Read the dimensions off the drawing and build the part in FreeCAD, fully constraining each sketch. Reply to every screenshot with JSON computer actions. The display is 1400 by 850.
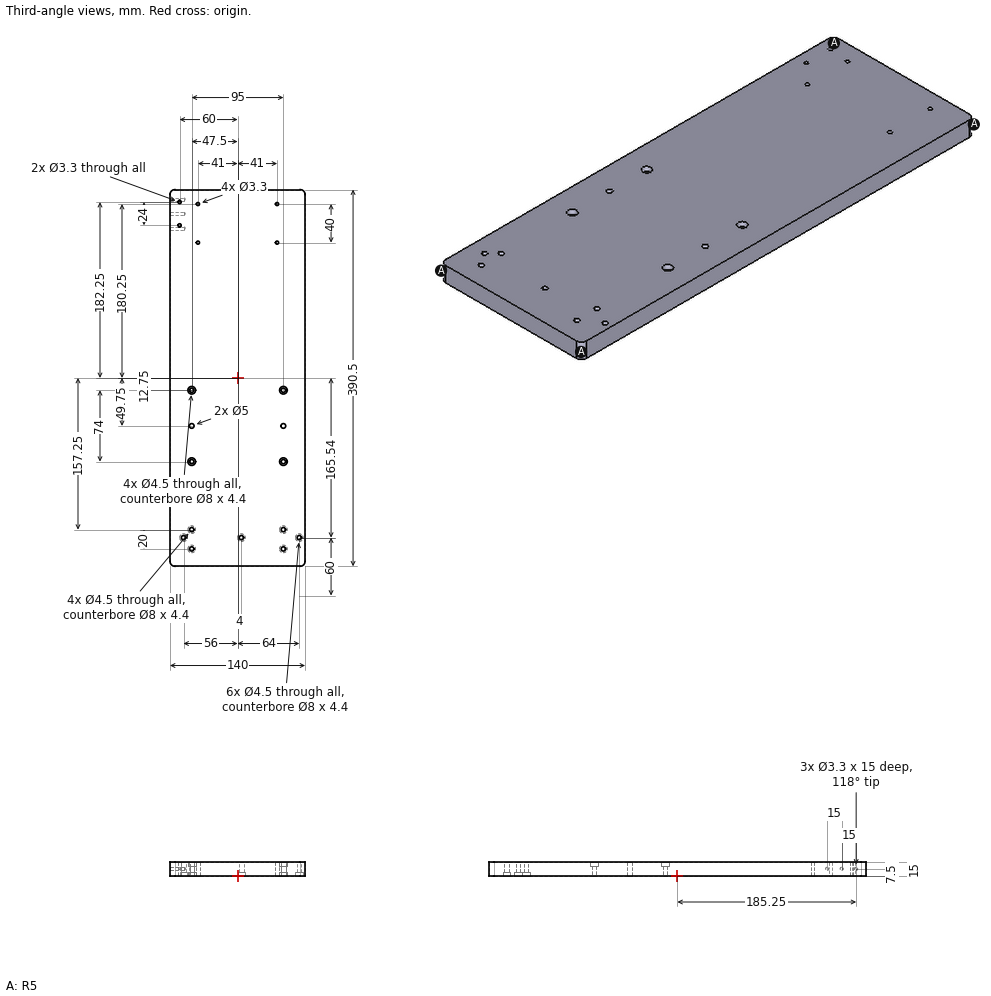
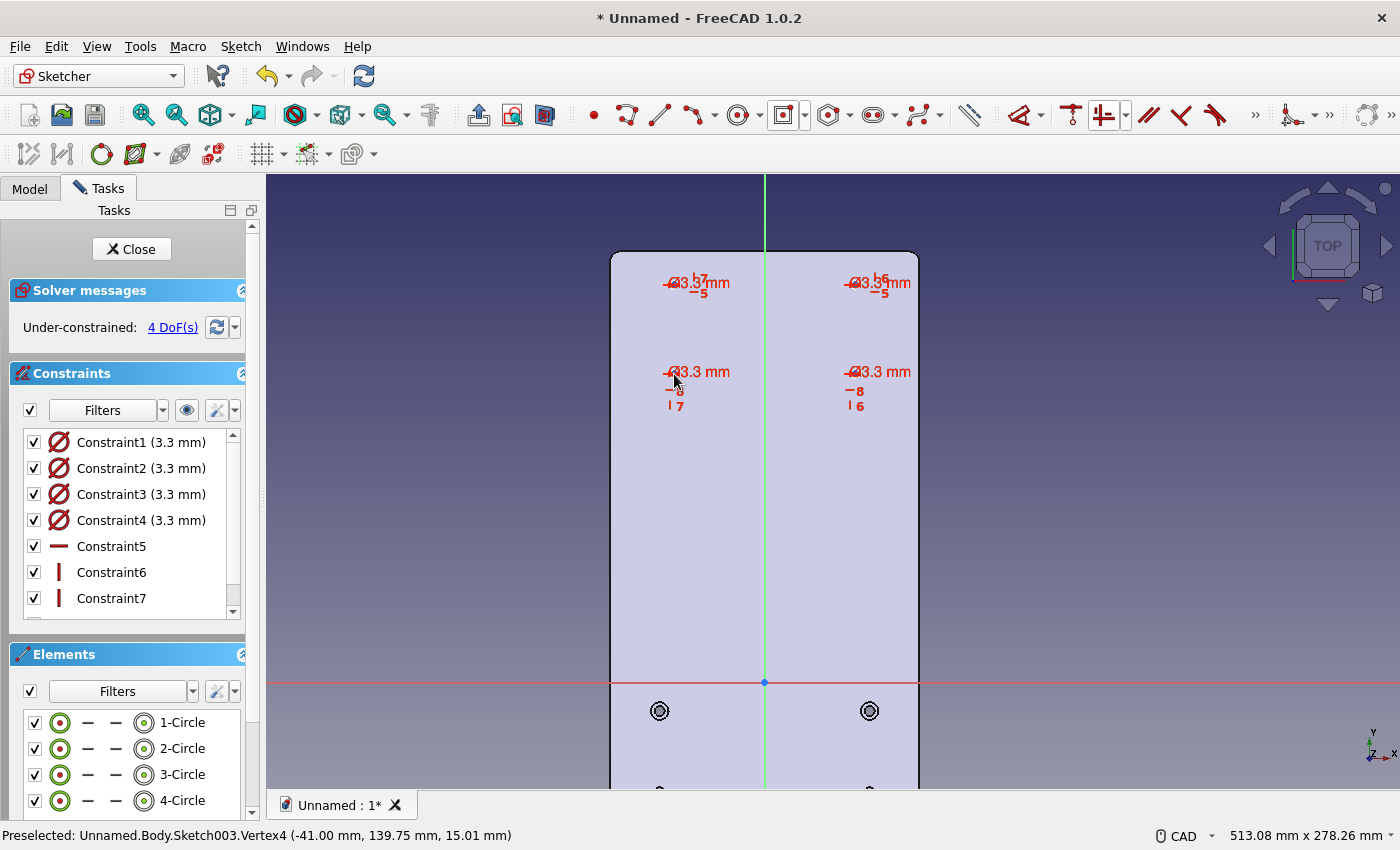
{"action": "left_click", "coordinate": [1018, 116]}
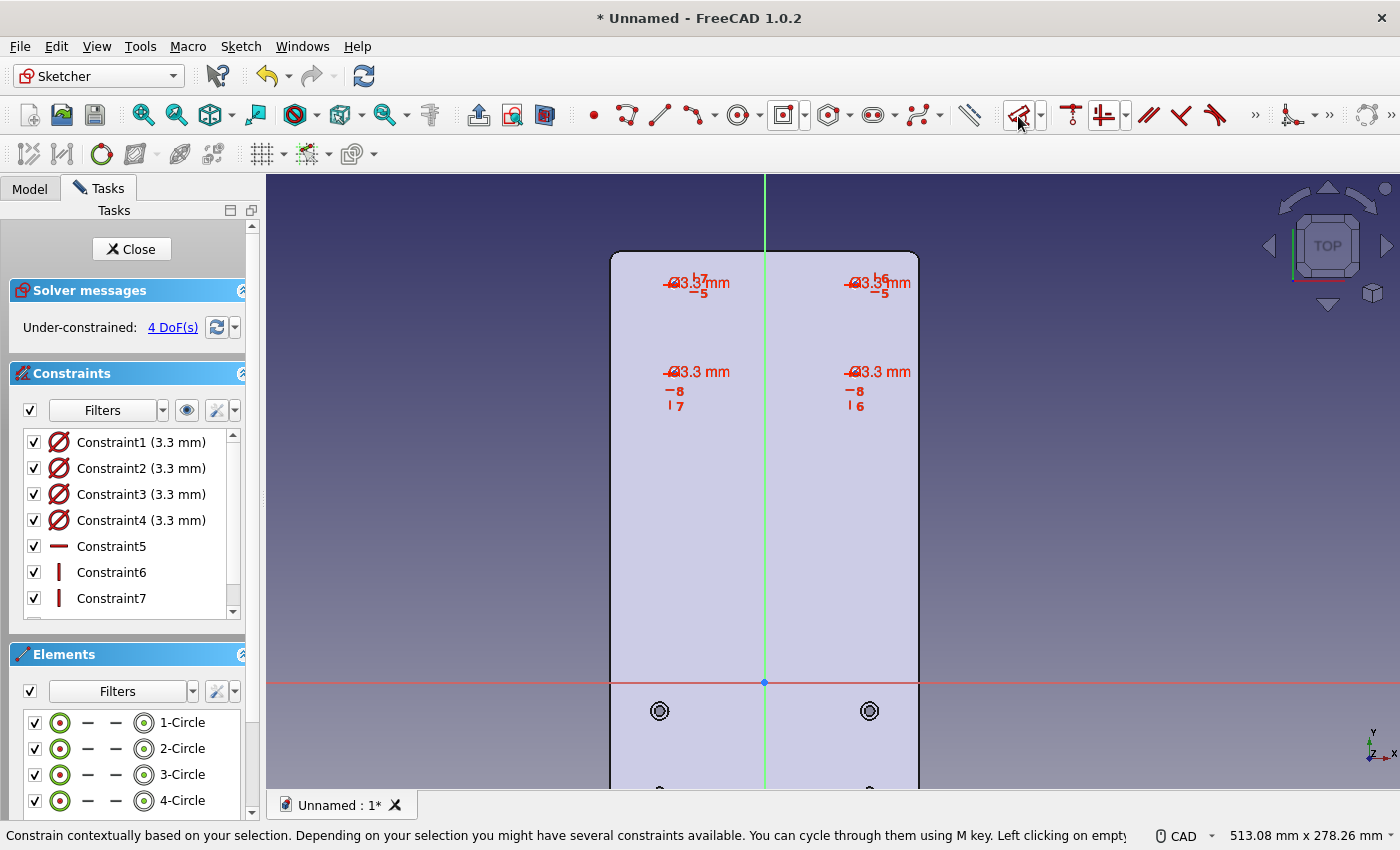
{"action": "left_click", "coordinate": [674, 285]}
{"action": "left_click", "coordinate": [719, 717]}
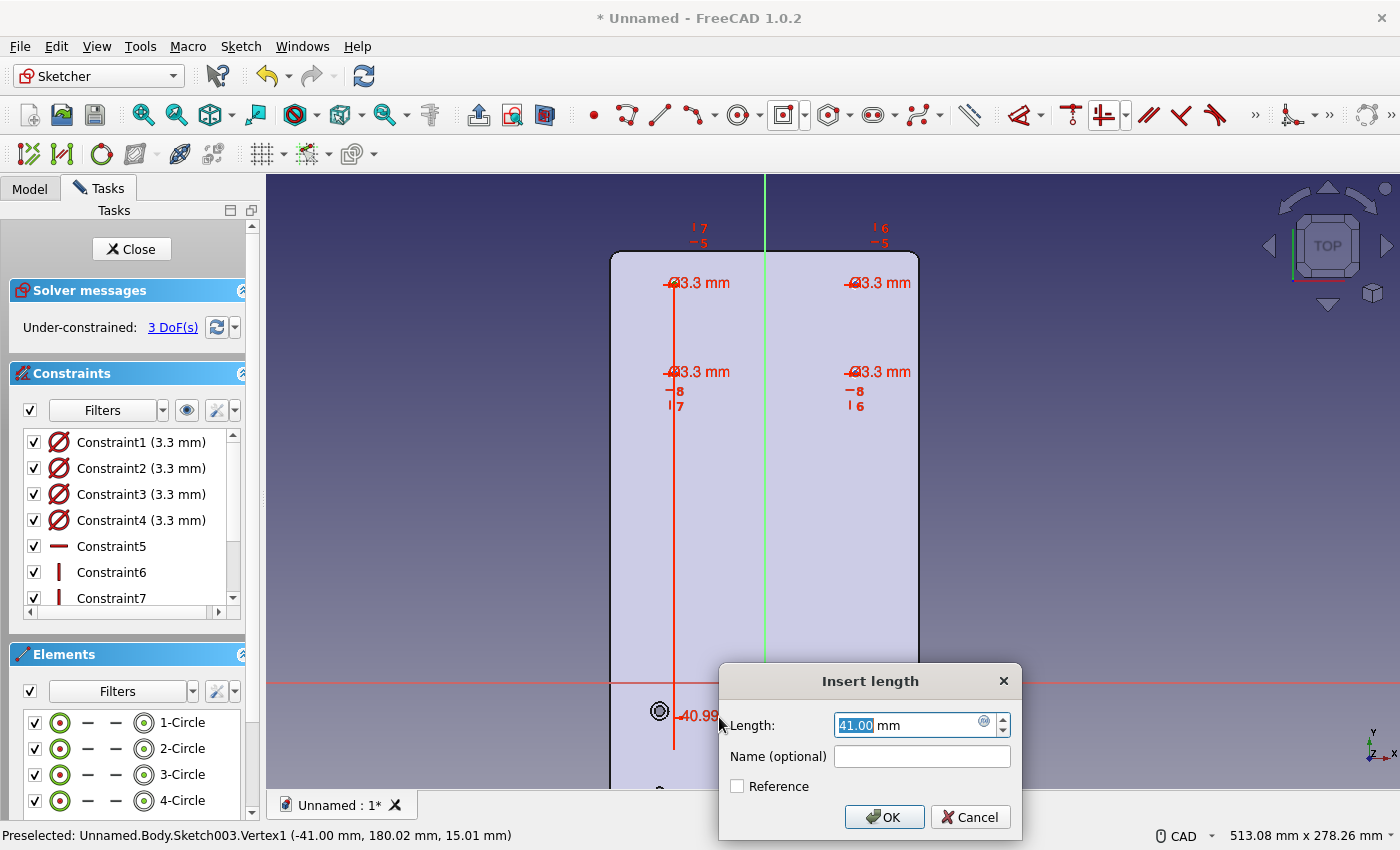
{"action": "type", "text": "41"}
{"action": "key", "text": "Return"}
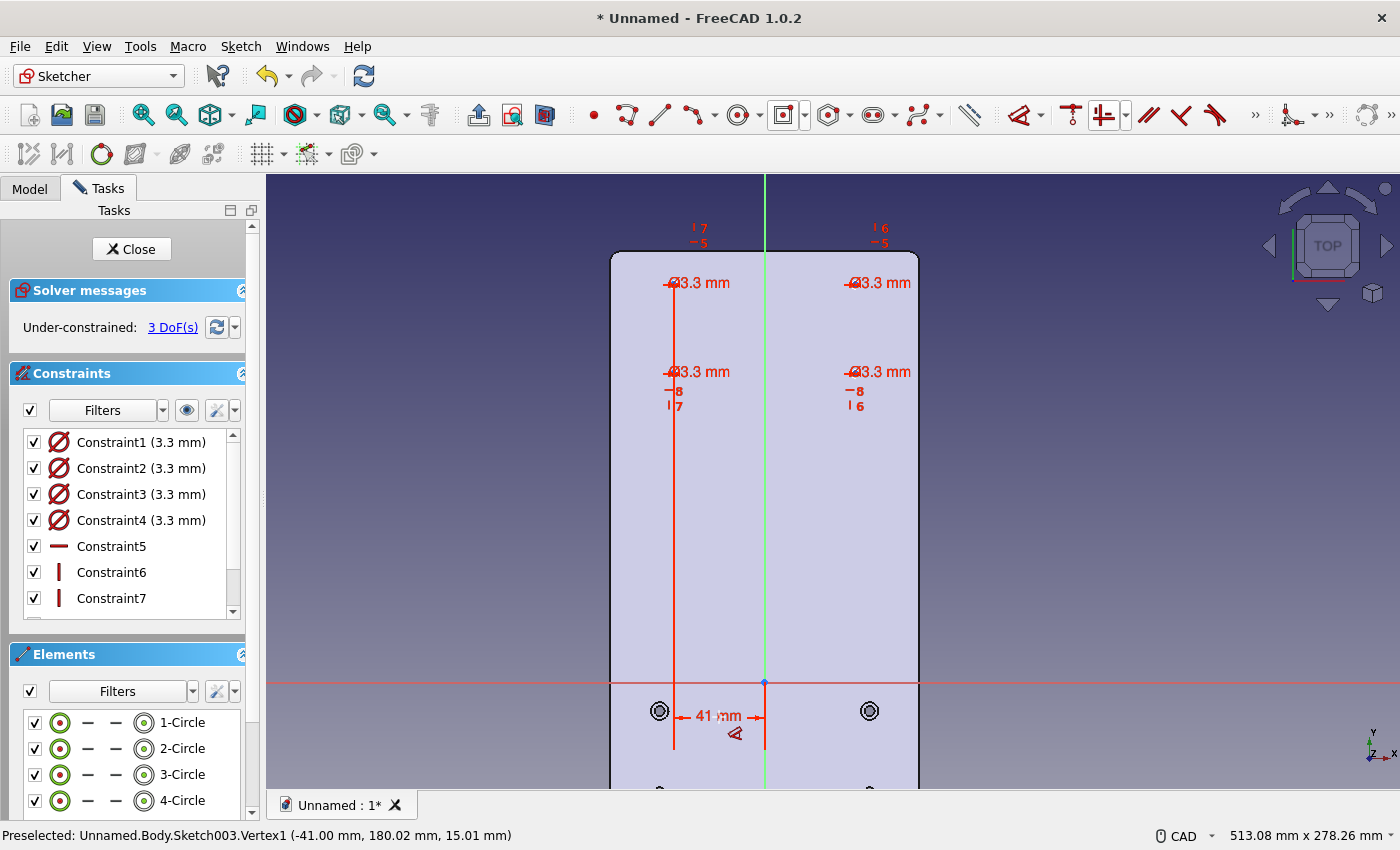
{"action": "left_click", "coordinate": [855, 285]}
{"action": "left_click", "coordinate": [810, 717]}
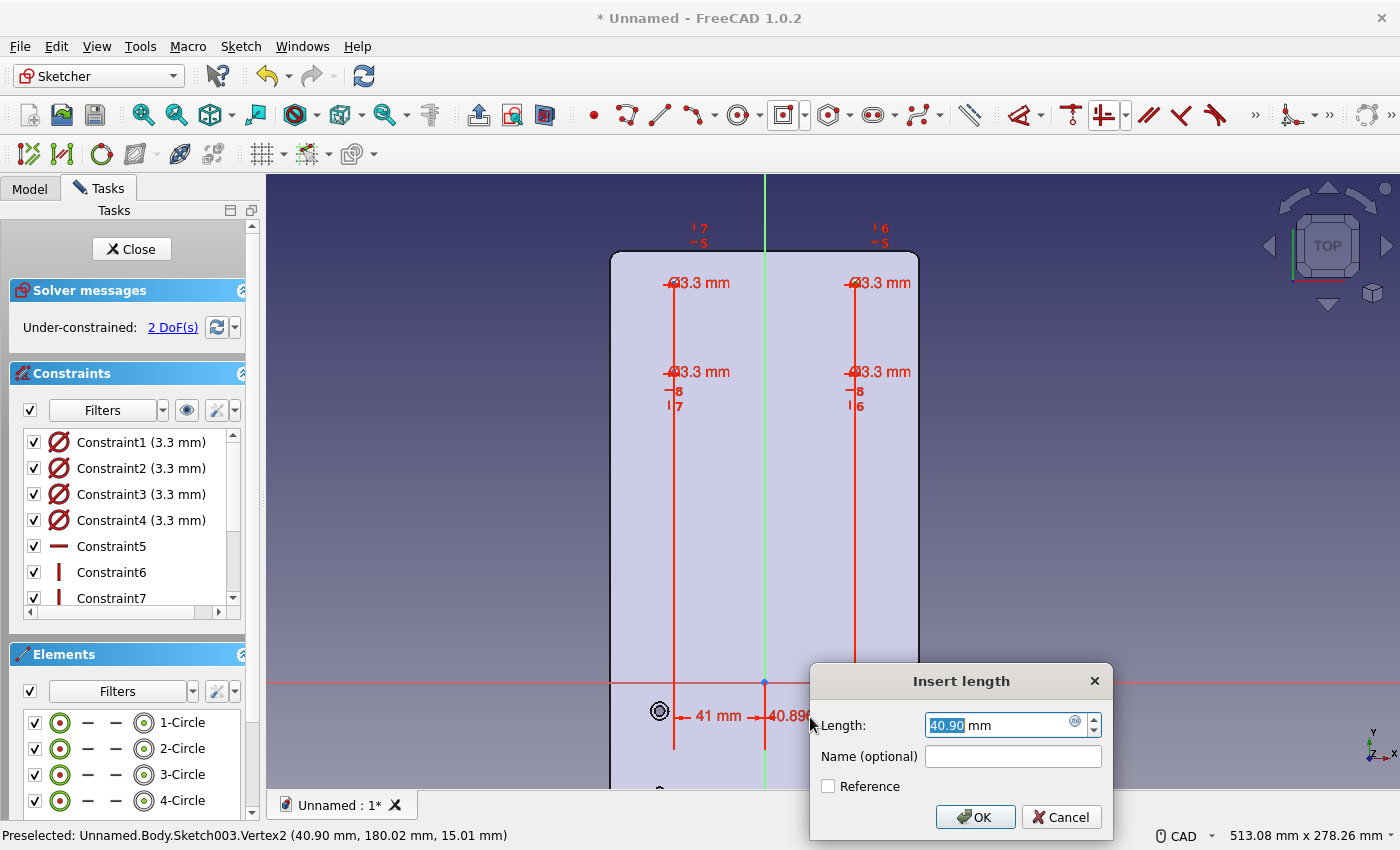
{"action": "type", "text": "41"}
{"action": "key", "text": "Return"}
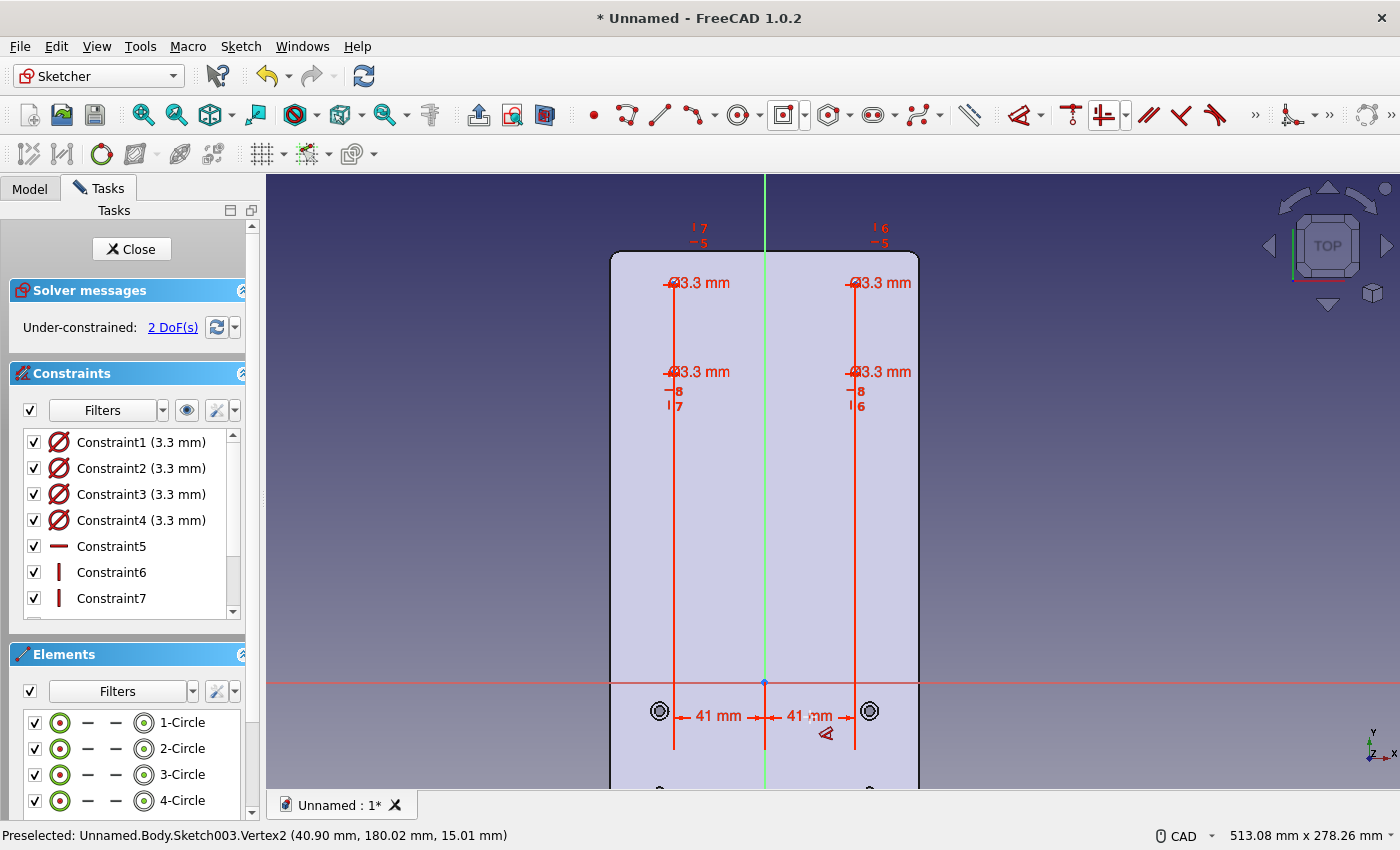
{"action": "left_click", "coordinate": [855, 285]}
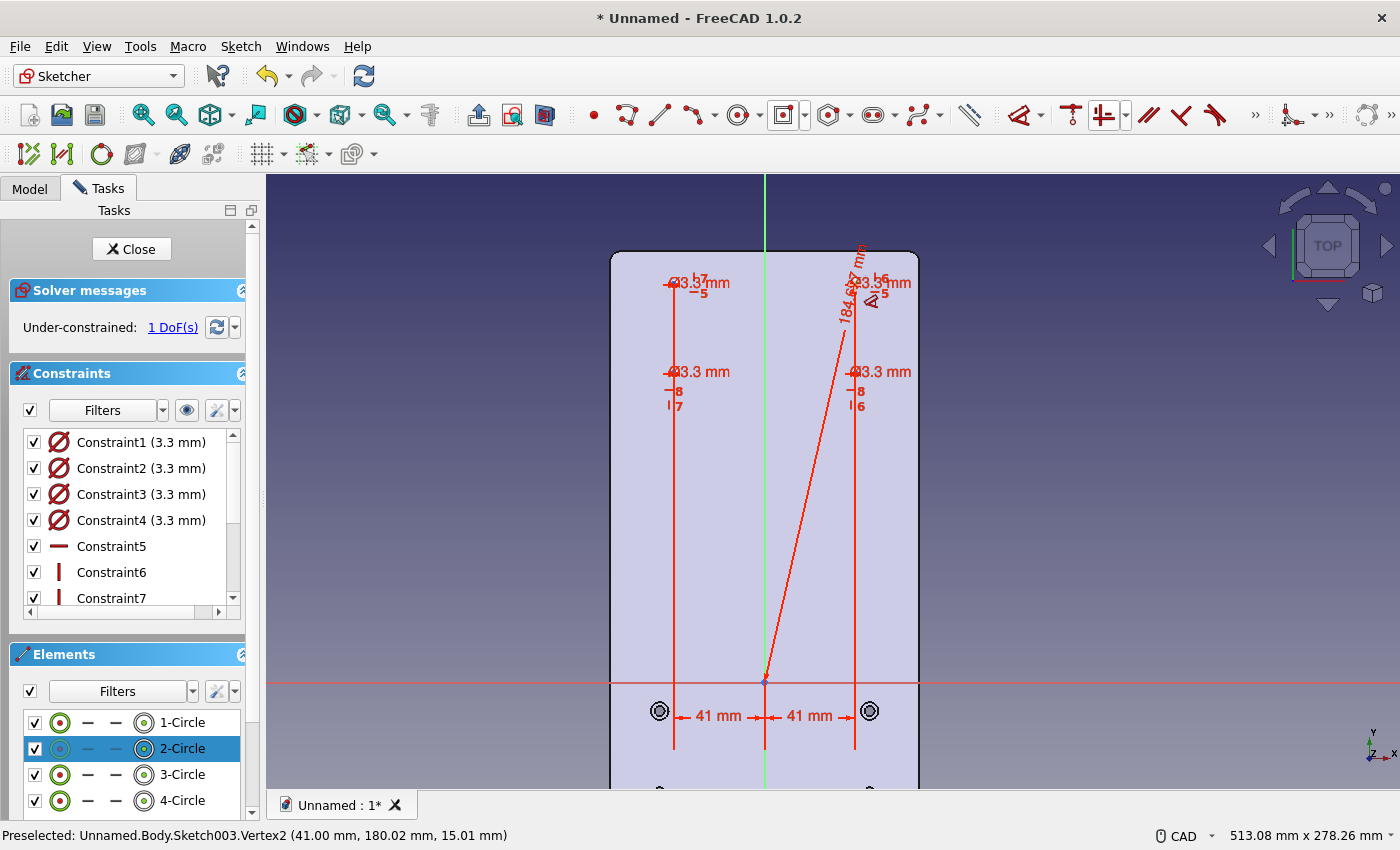
{"action": "left_click", "coordinate": [855, 374]}
{"action": "left_click", "coordinate": [889, 330]}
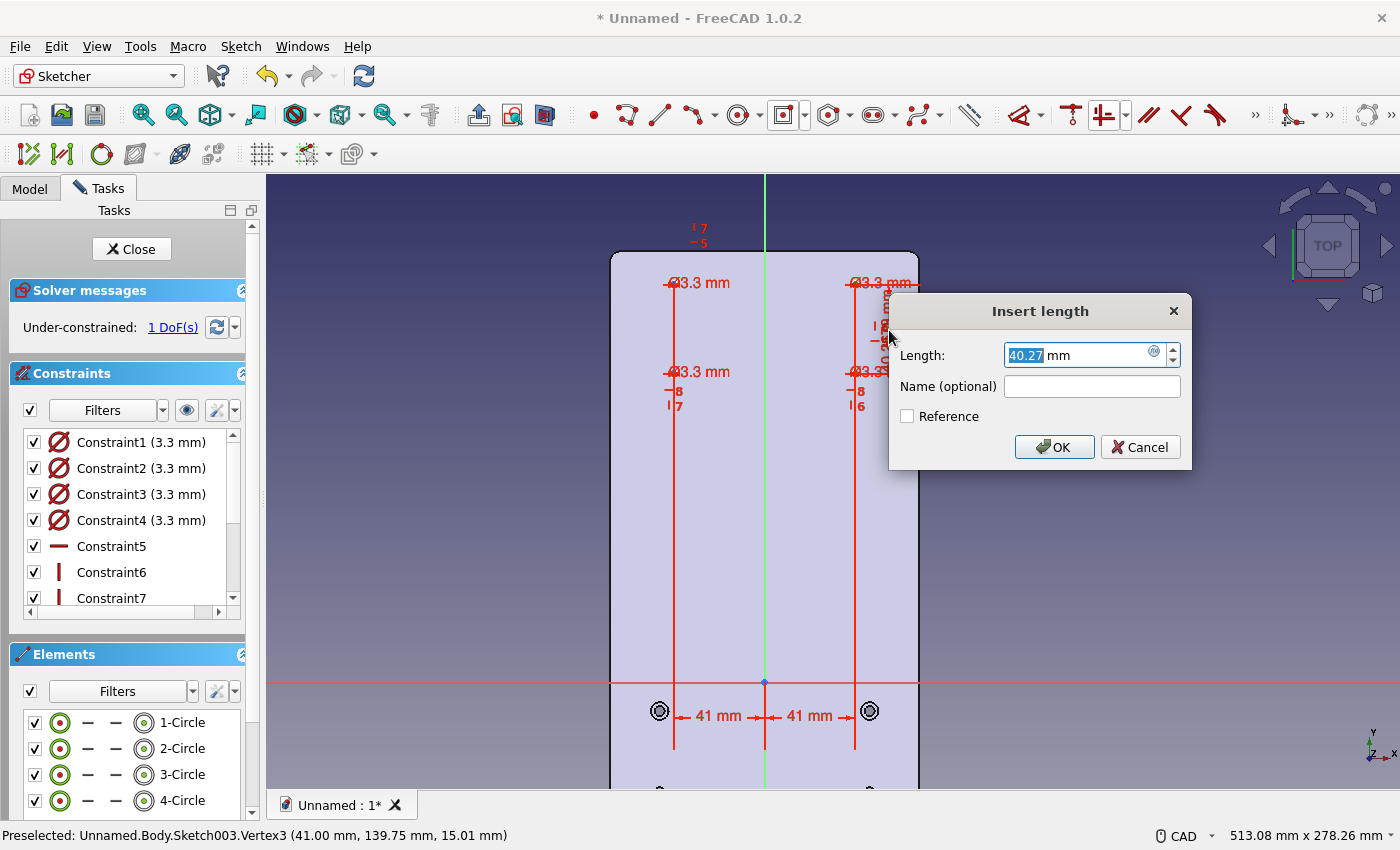
{"action": "type", "text": "40"}
{"action": "key", "text": "Return"}